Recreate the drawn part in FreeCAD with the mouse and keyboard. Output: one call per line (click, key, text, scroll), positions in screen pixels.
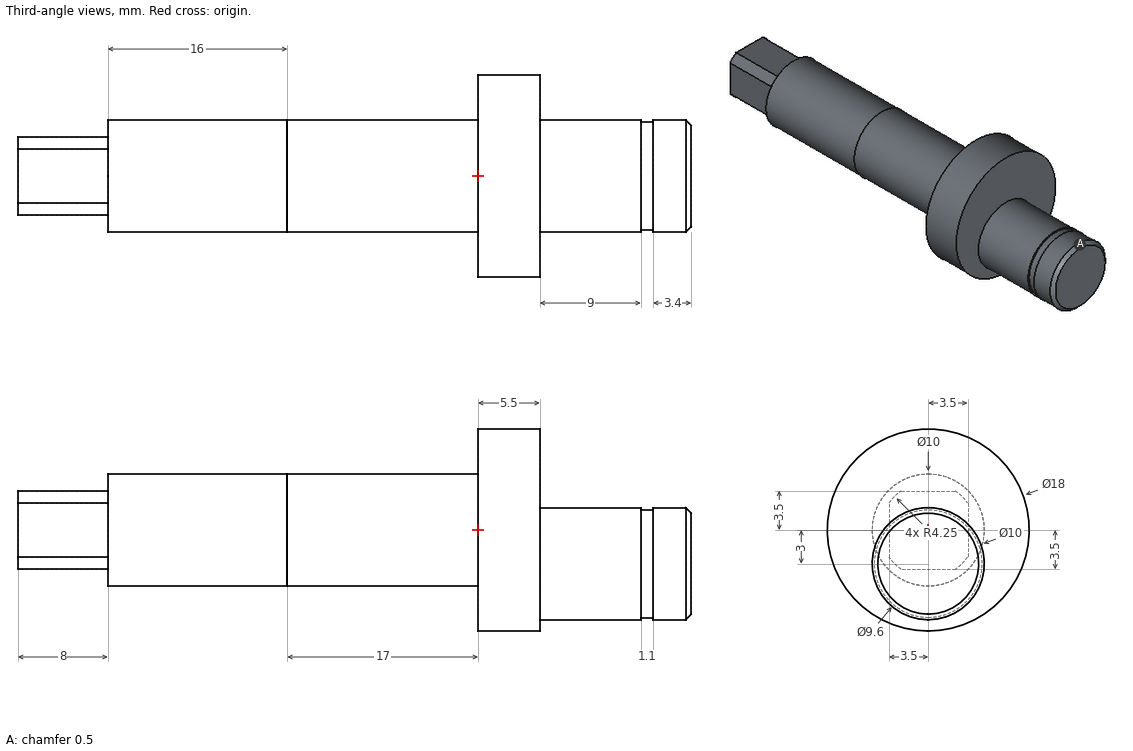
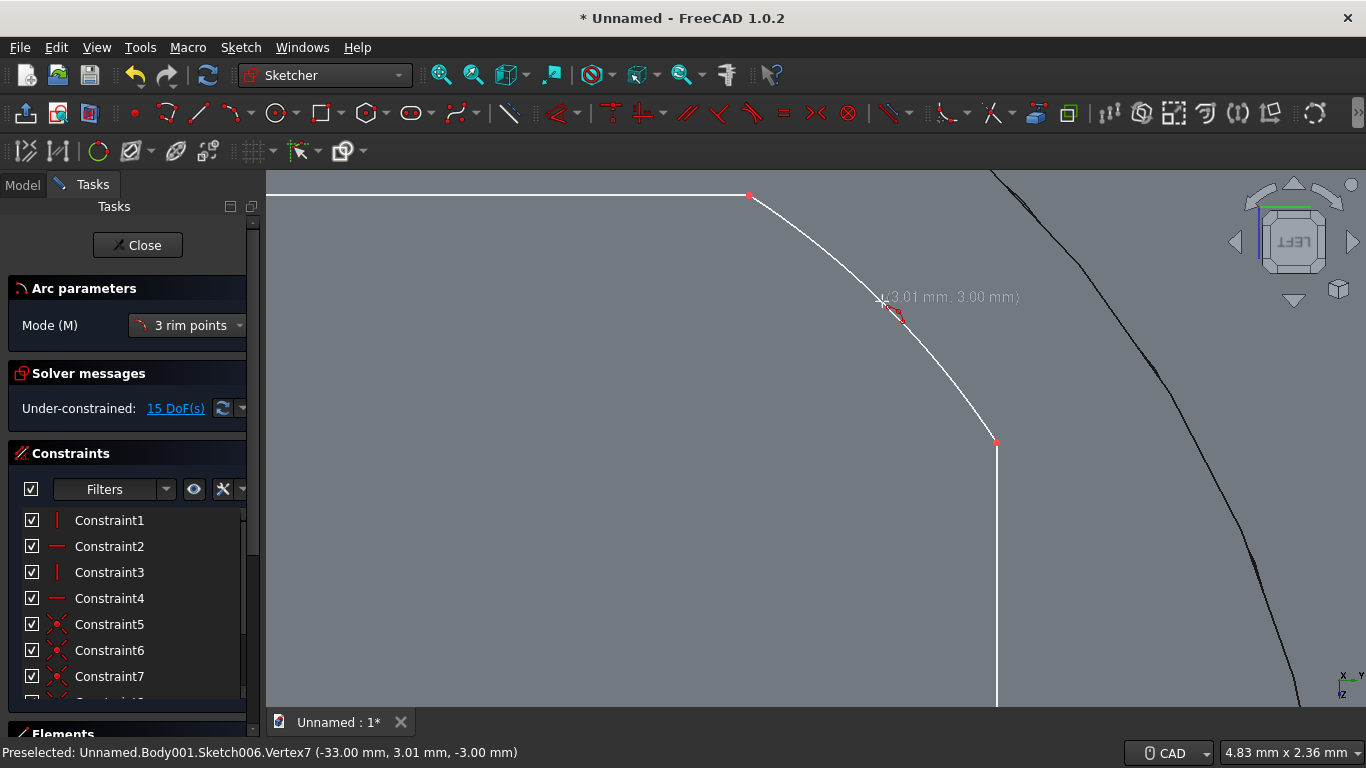
scroll(886, 300, down, 8)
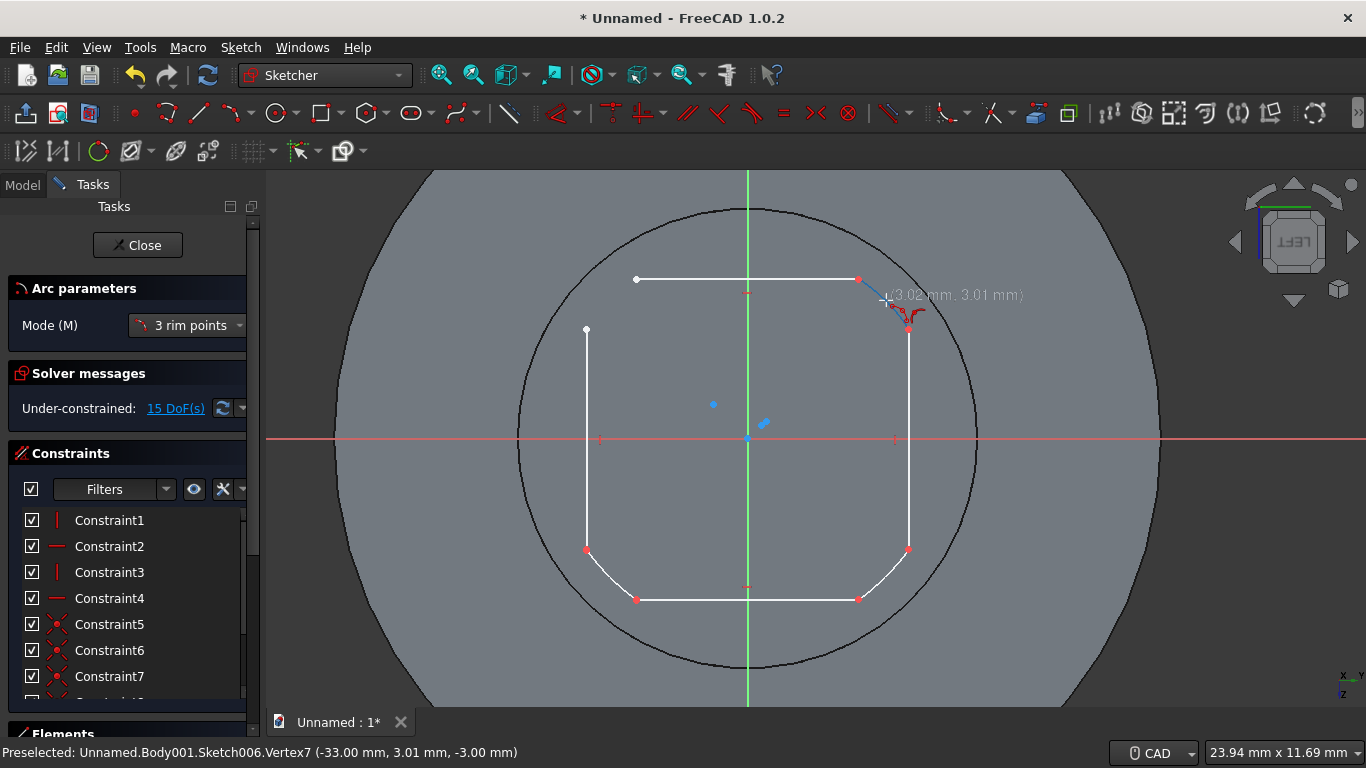
click(637, 279)
click(587, 329)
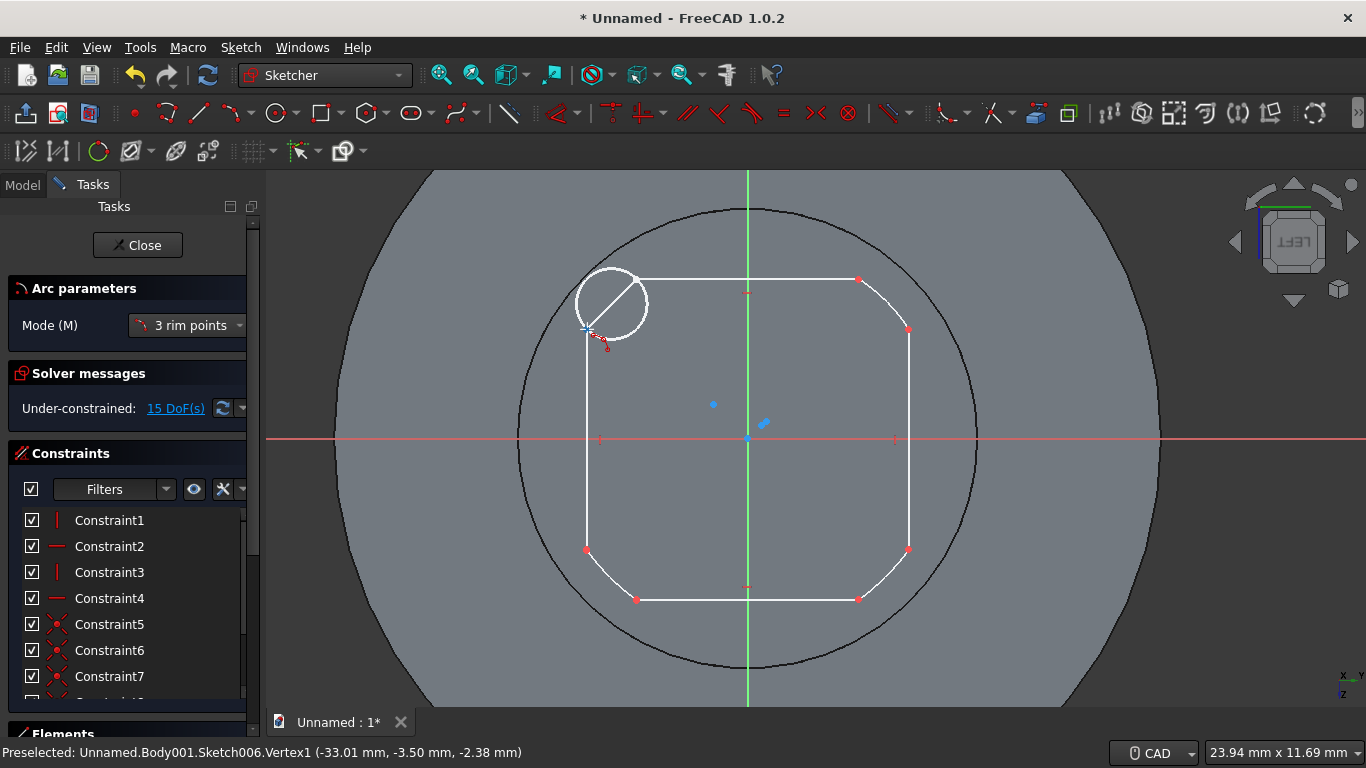
scroll(609, 300, up, 8)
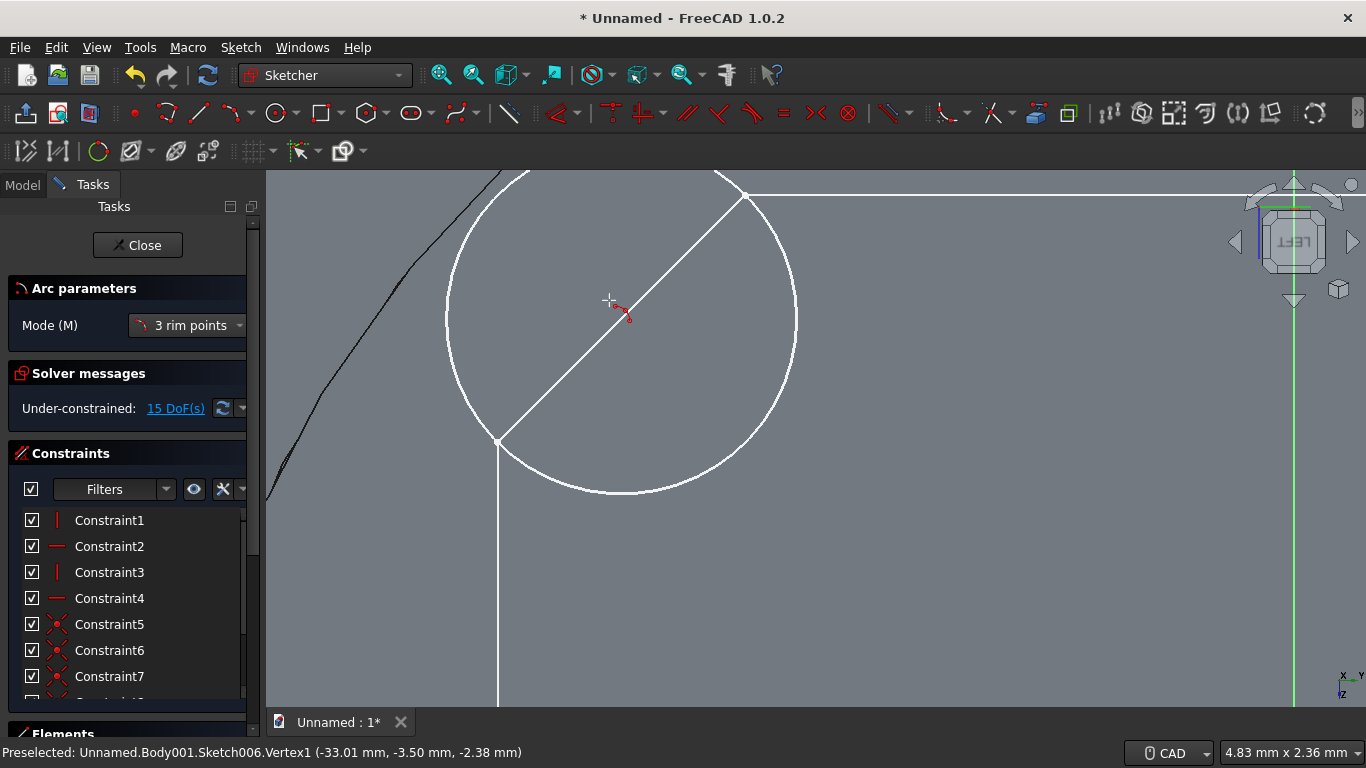
click(610, 301)
key(Escape)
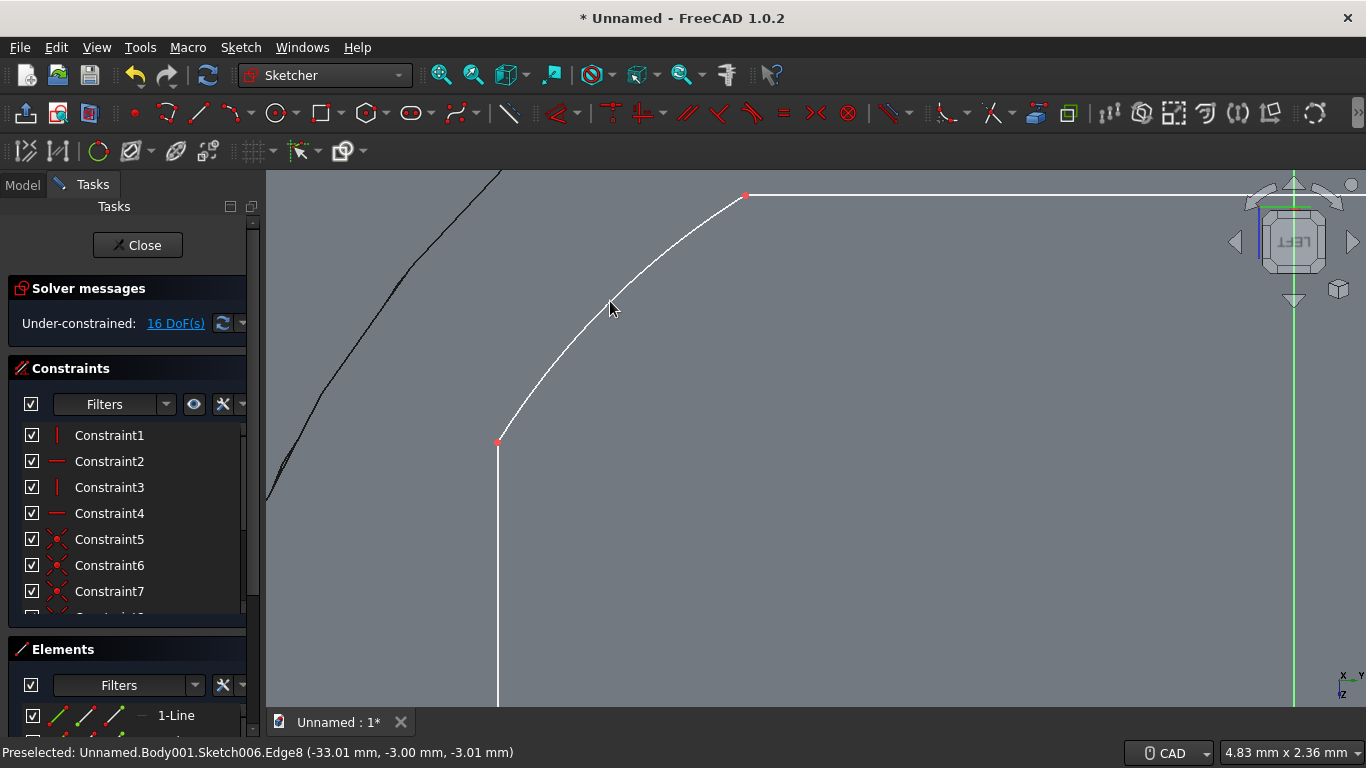
scroll(609, 300, down, 8)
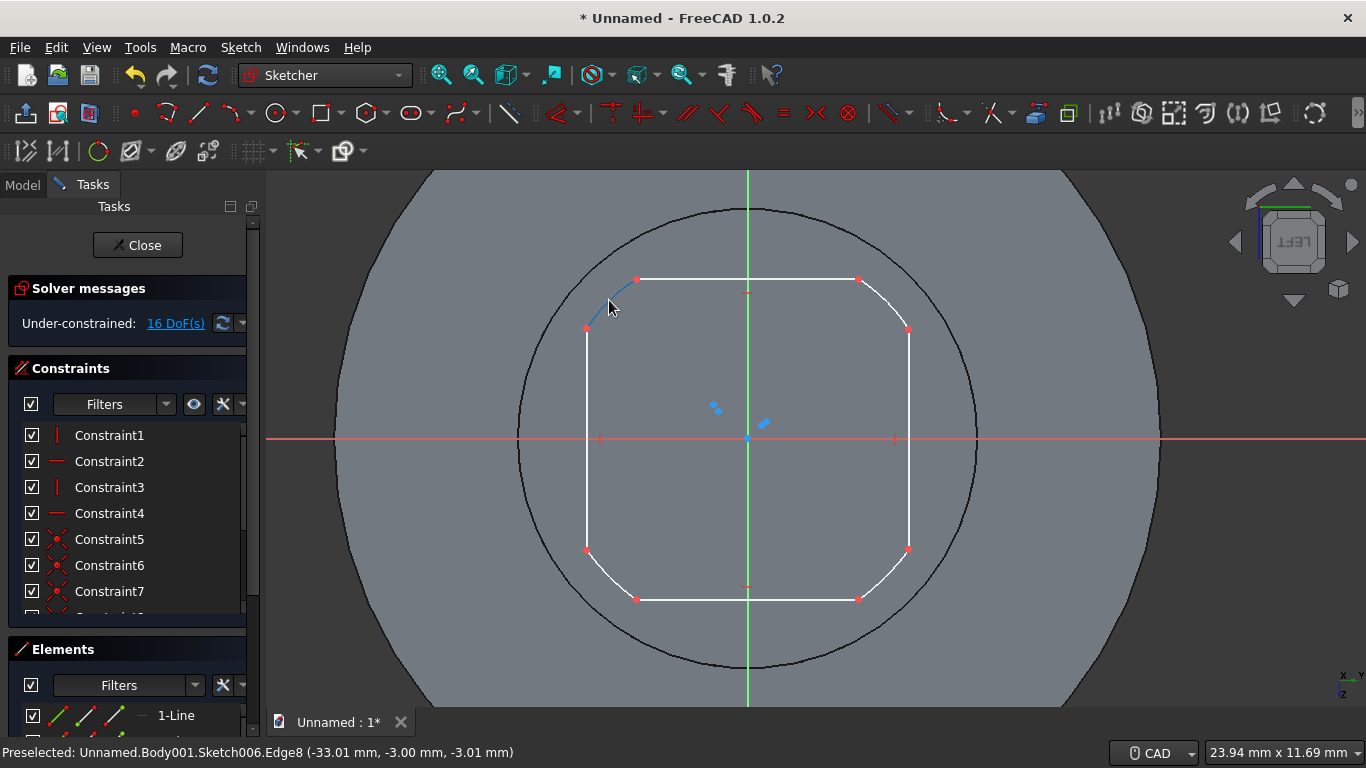
click(600, 567)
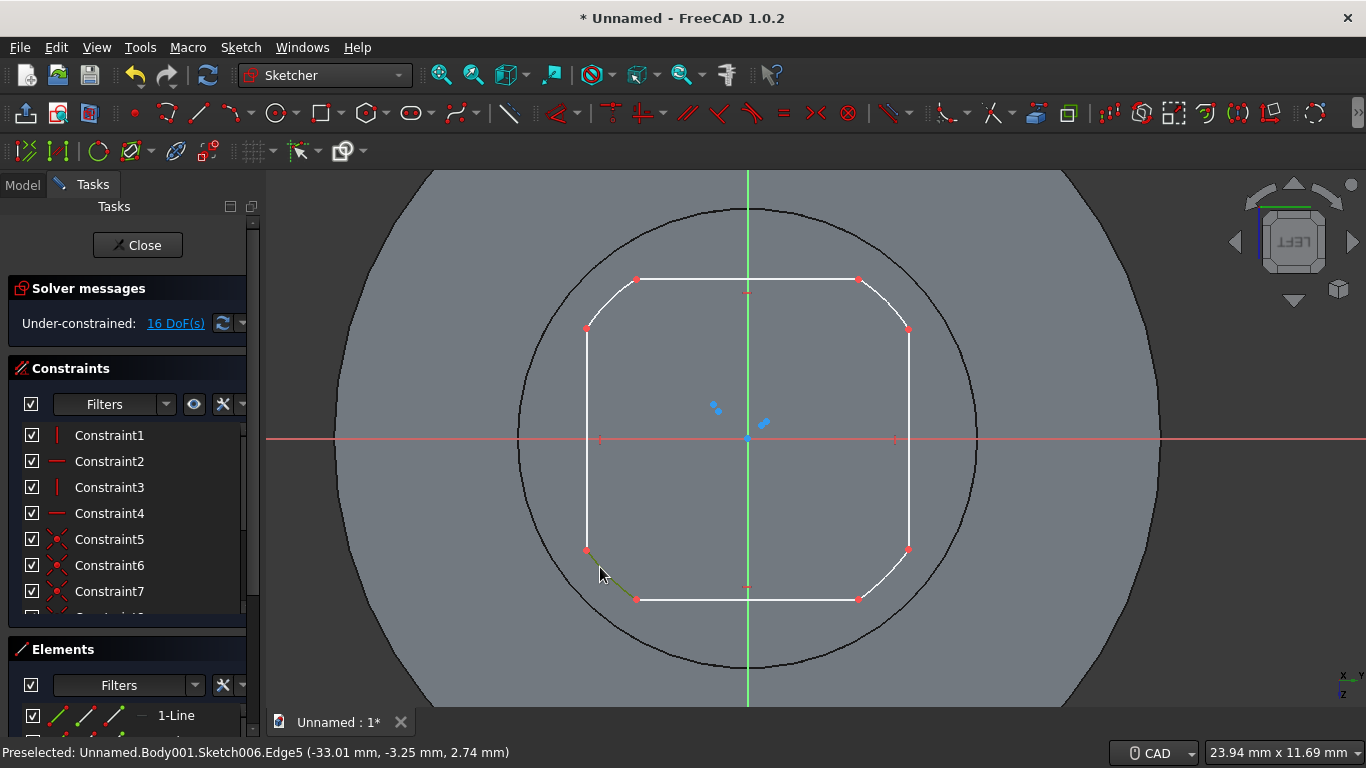
click(875, 587)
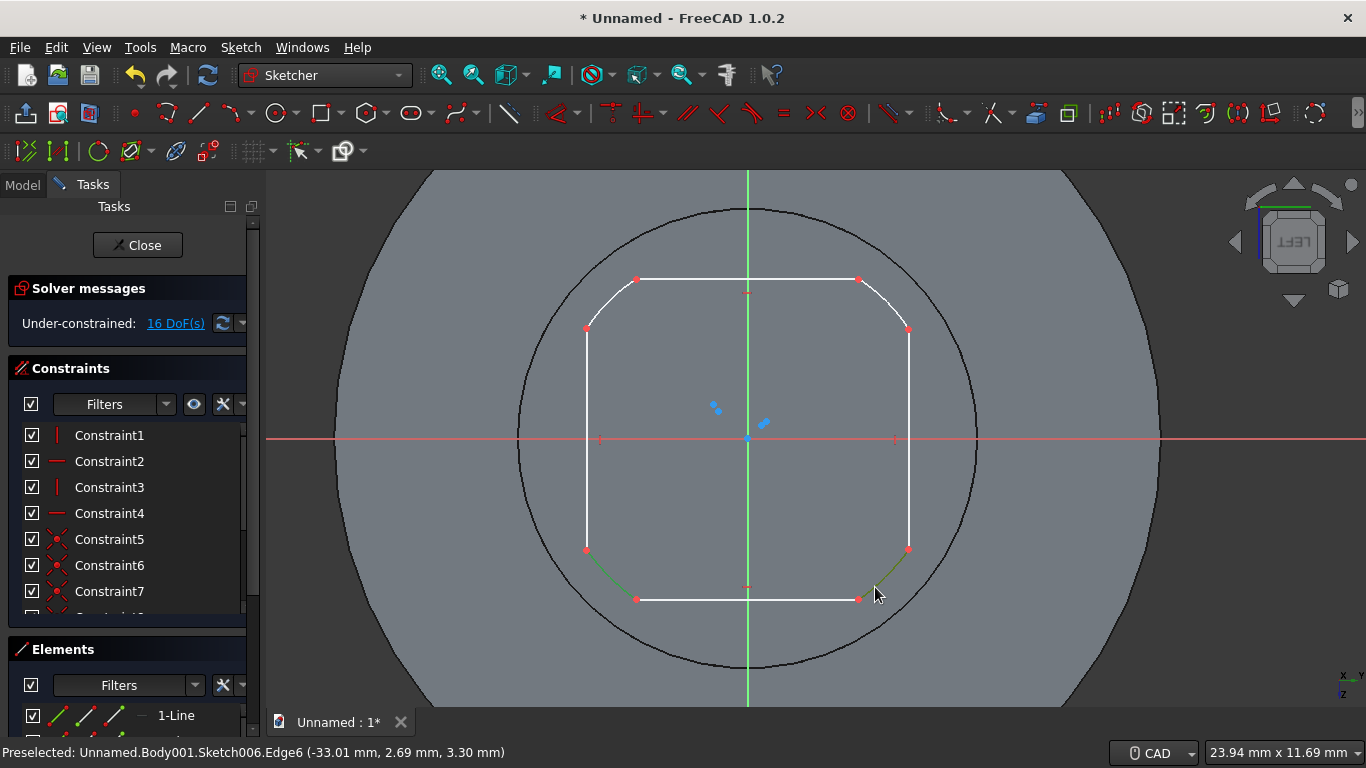
key(c)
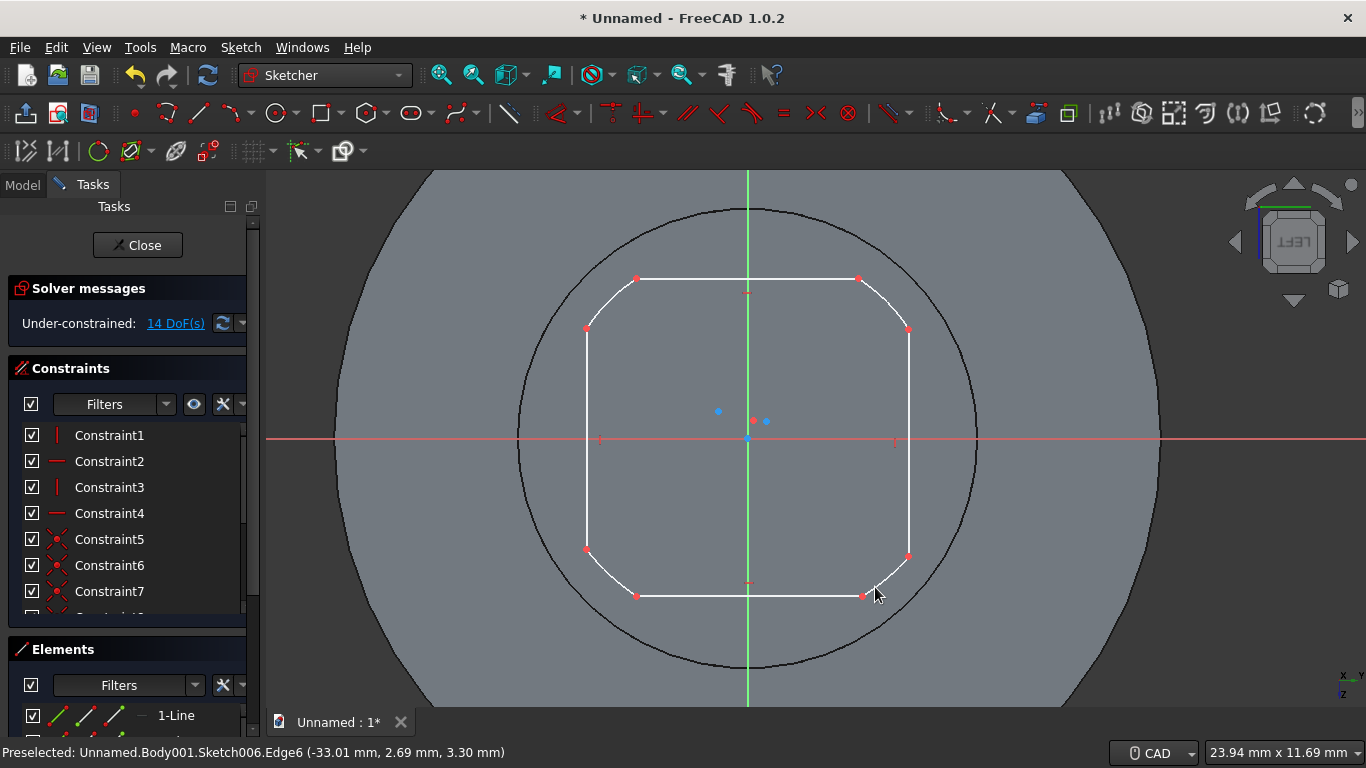
click(600, 565)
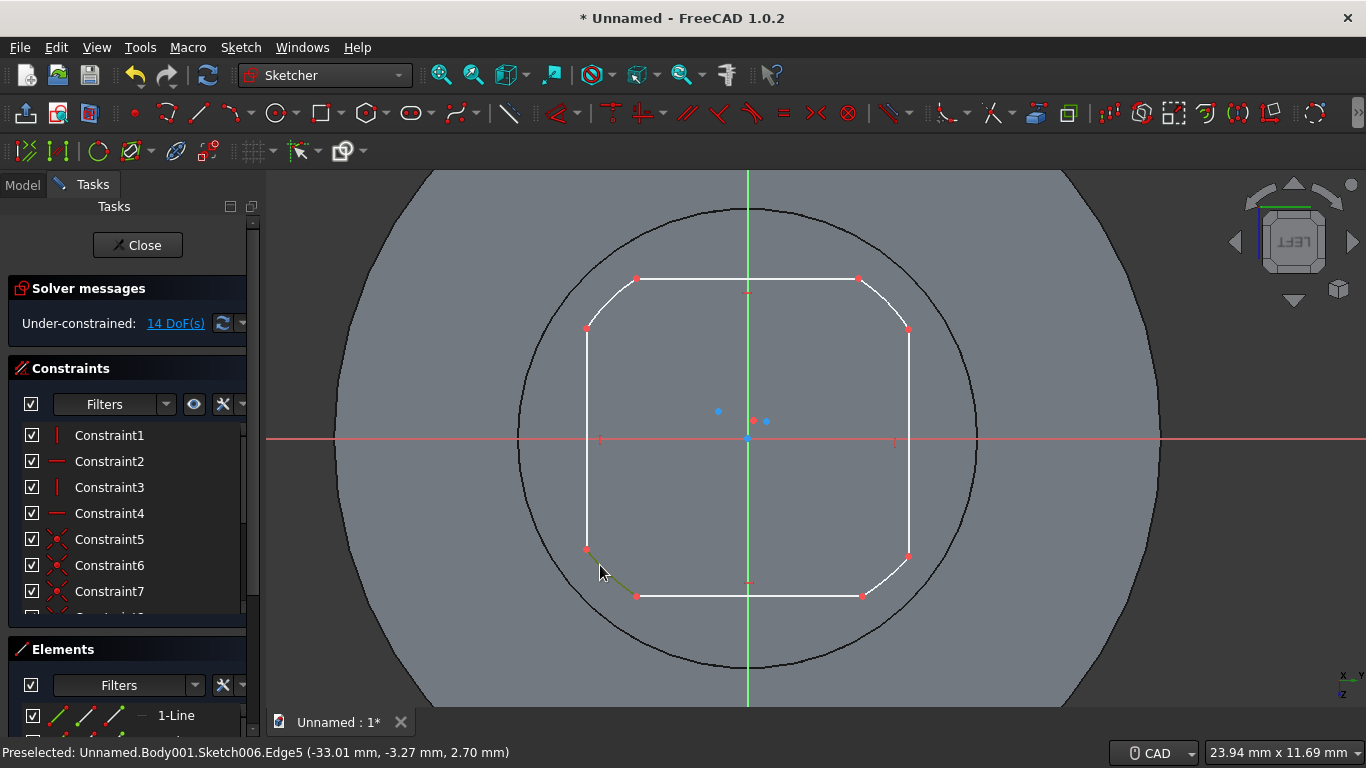
click(896, 312)